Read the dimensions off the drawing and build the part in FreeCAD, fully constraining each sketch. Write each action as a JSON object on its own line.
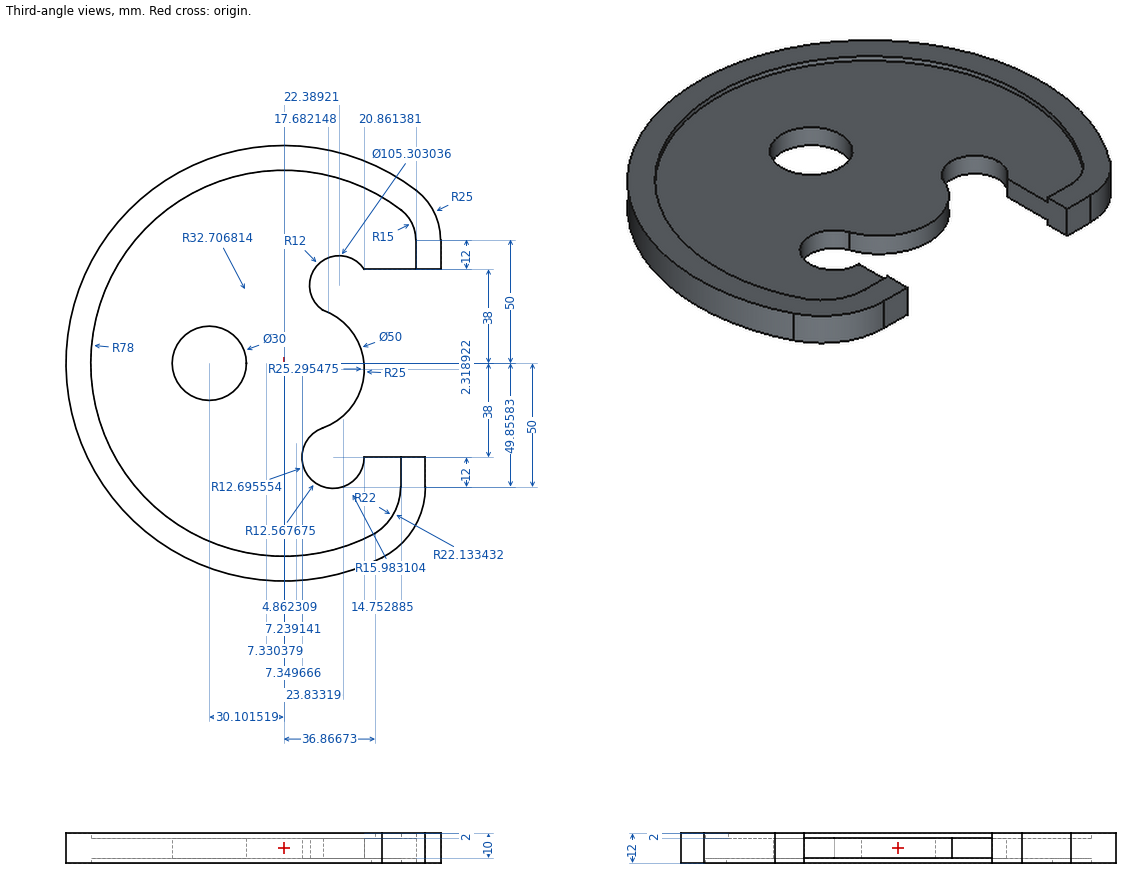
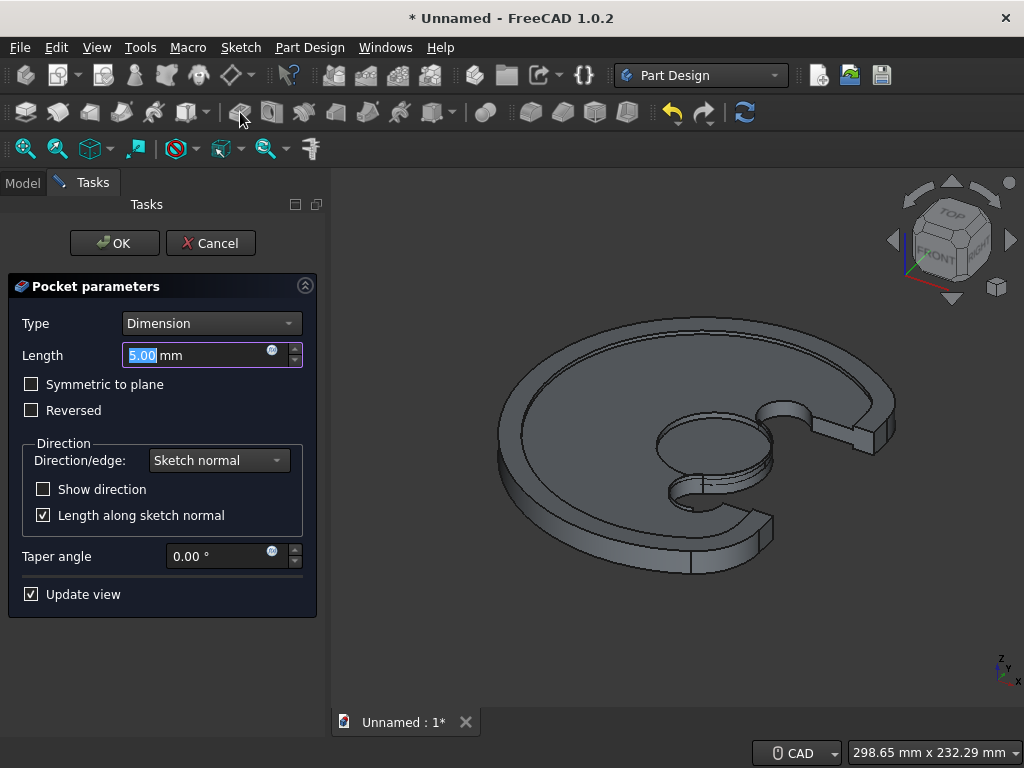
{"action": "type", "text": "2"}
{"action": "key", "text": "Tab"}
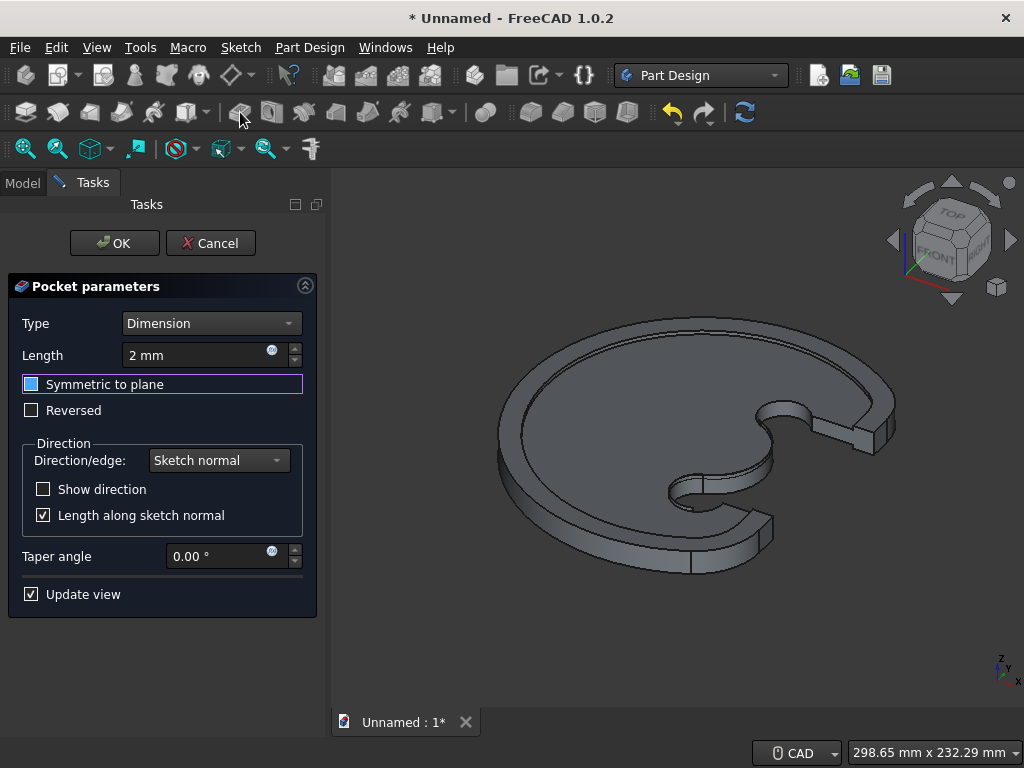
{"action": "left_click", "coordinate": [115, 243]}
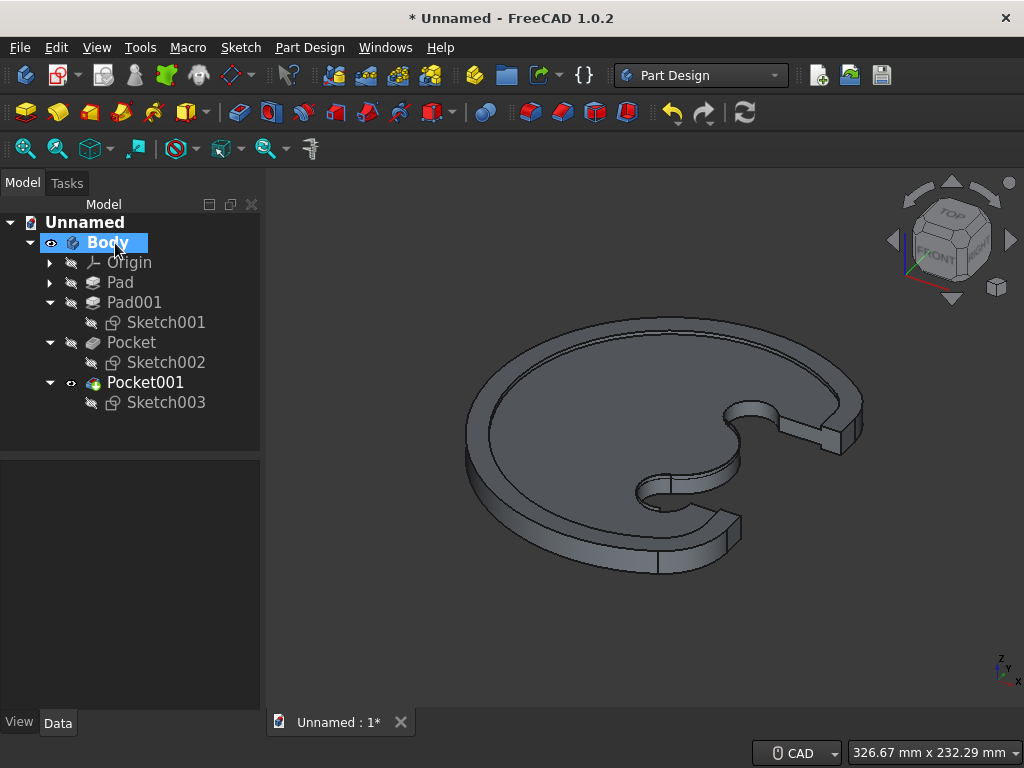
{"action": "left_click", "coordinate": [607, 416]}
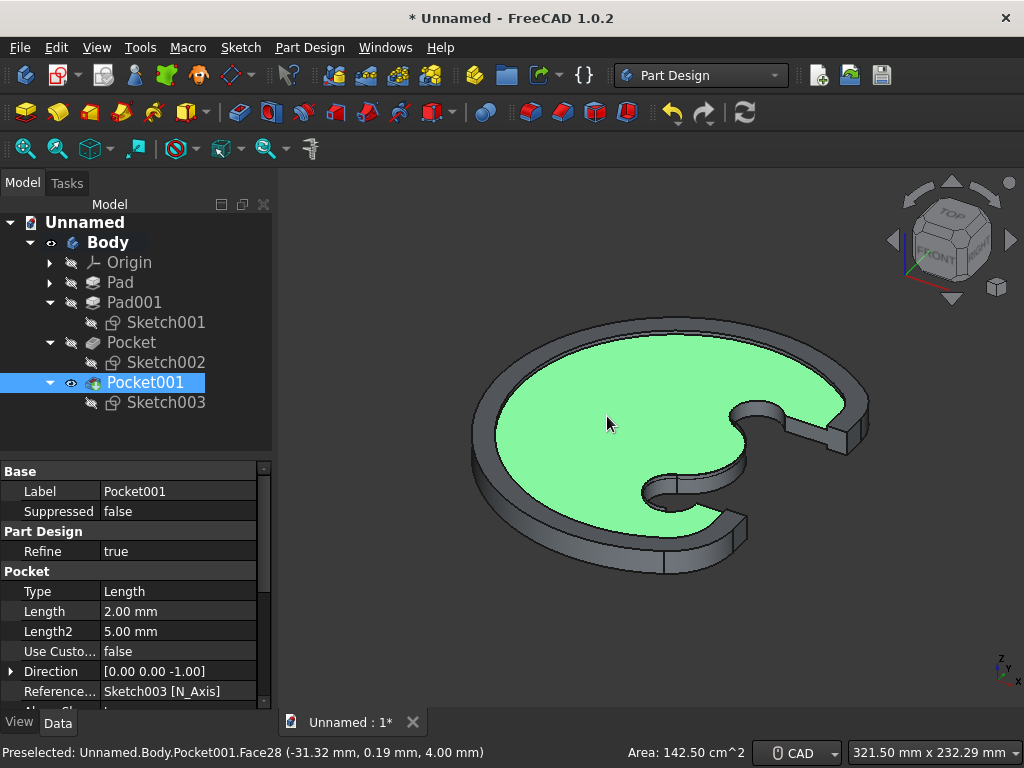
{"action": "left_click", "coordinate": [58, 76]}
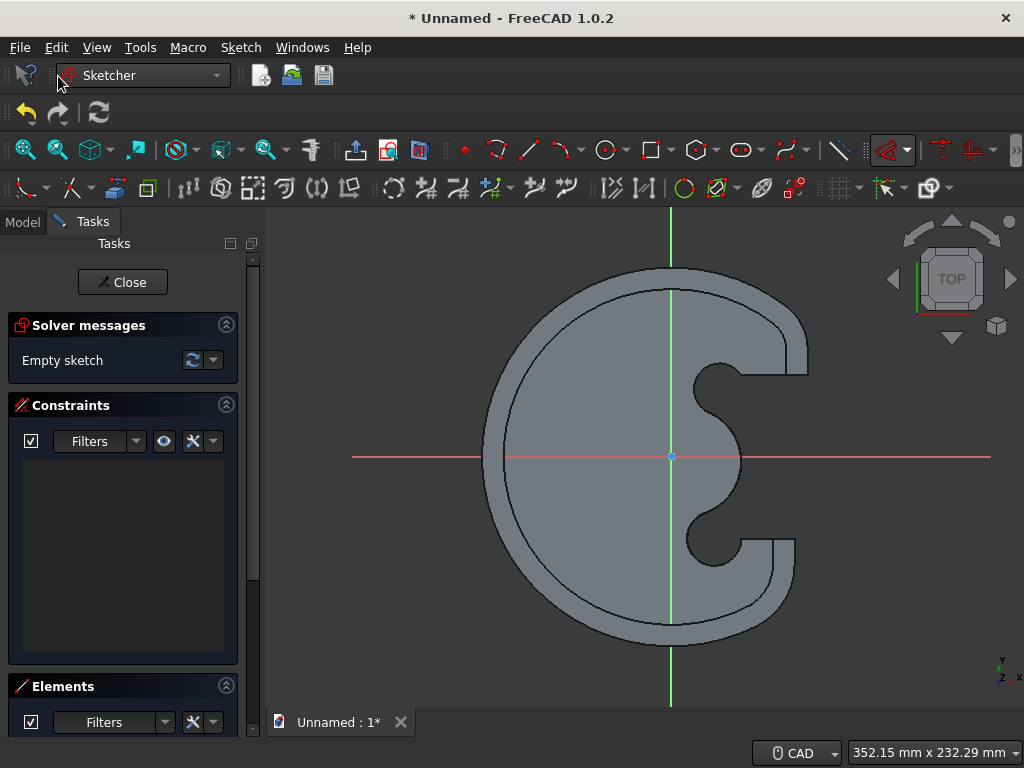
{"action": "scroll", "coordinate": [816, 512], "scroll_direction": "up", "scroll_amount": 3}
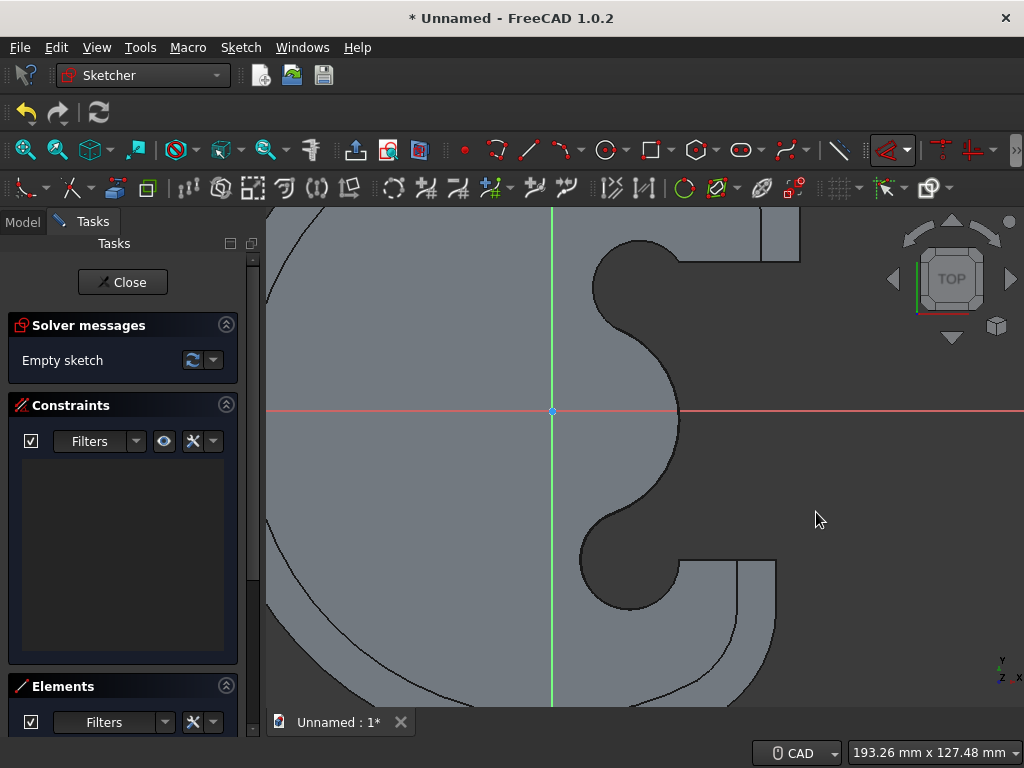
{"action": "key", "text": "g 3 a"}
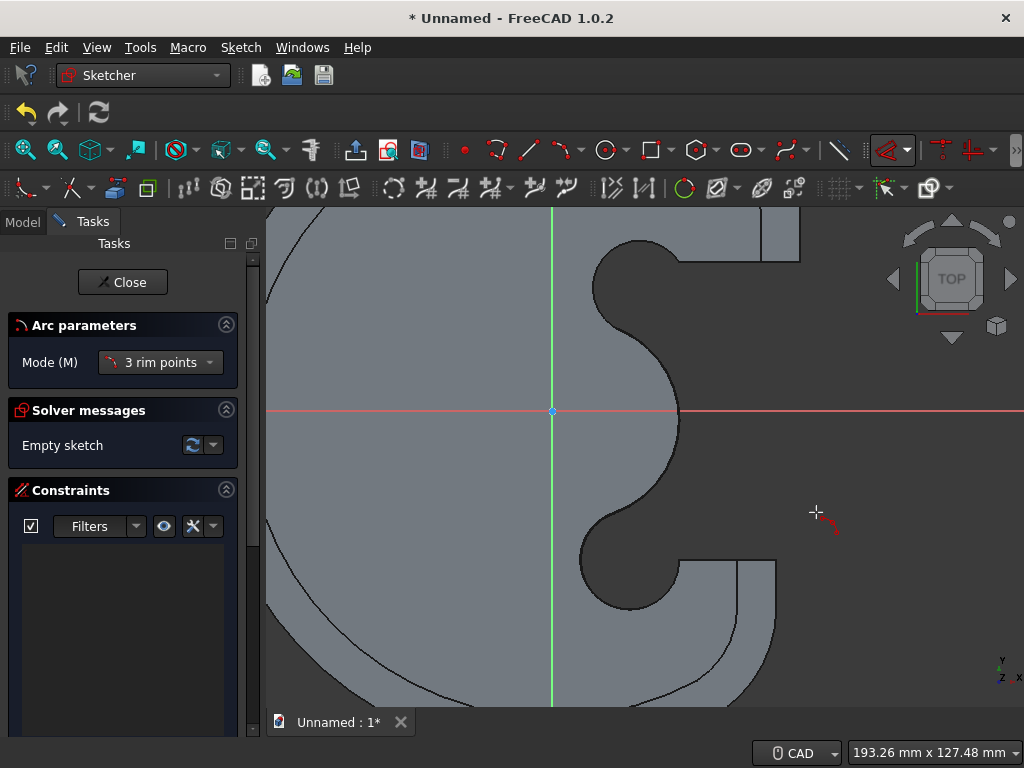
{"action": "left_click", "coordinate": [646, 499]}
{"action": "left_click", "coordinate": [571, 538]}
{"action": "left_click", "coordinate": [492, 298]}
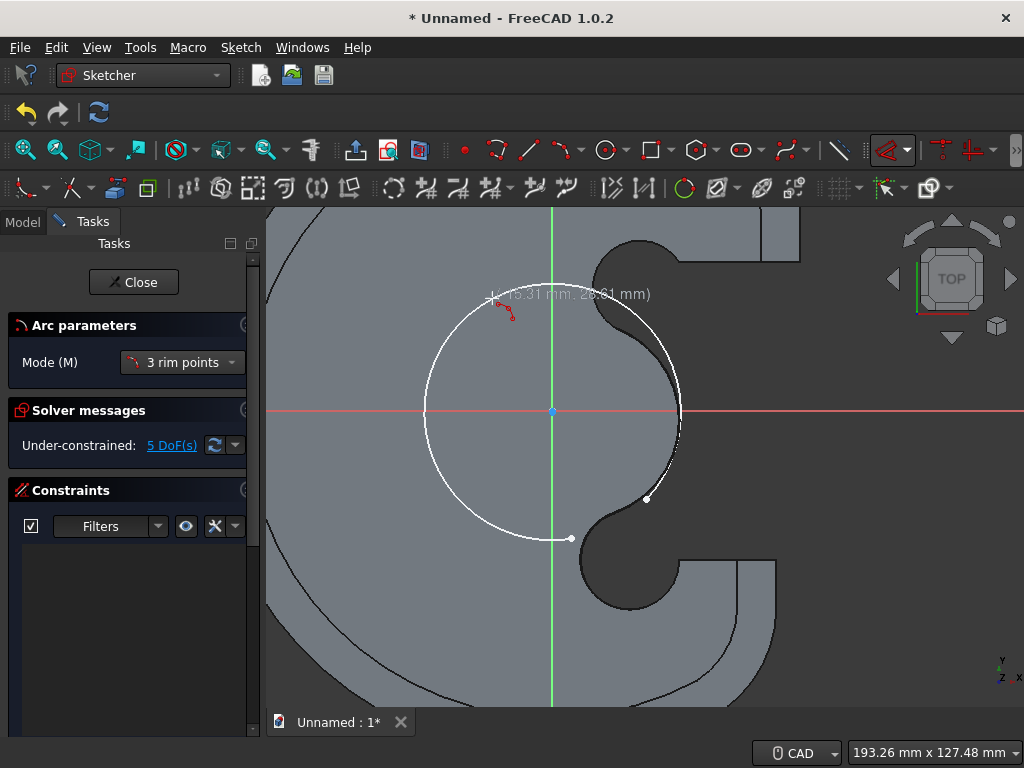
{"action": "left_click", "coordinate": [571, 539]}
{"action": "left_click", "coordinate": [646, 500]}
{"action": "left_click", "coordinate": [659, 615]}
{"action": "key", "text": "Escape"}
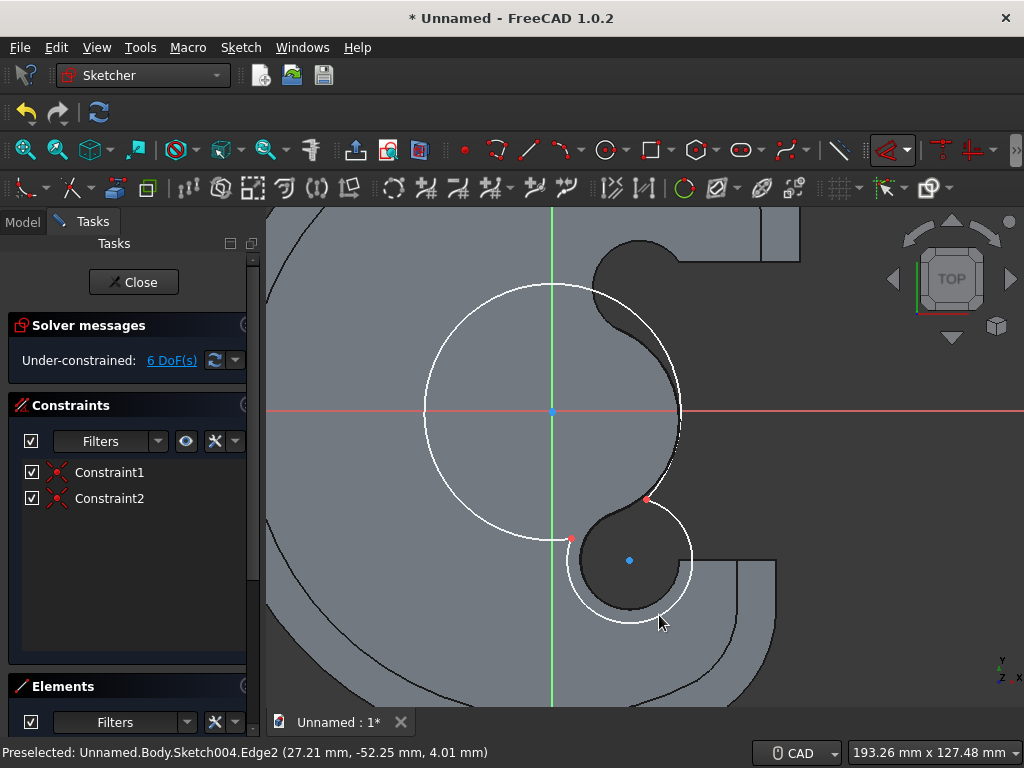
{"action": "left_click_drag", "start_coordinate": [542, 401], "coordinate": [563, 422]}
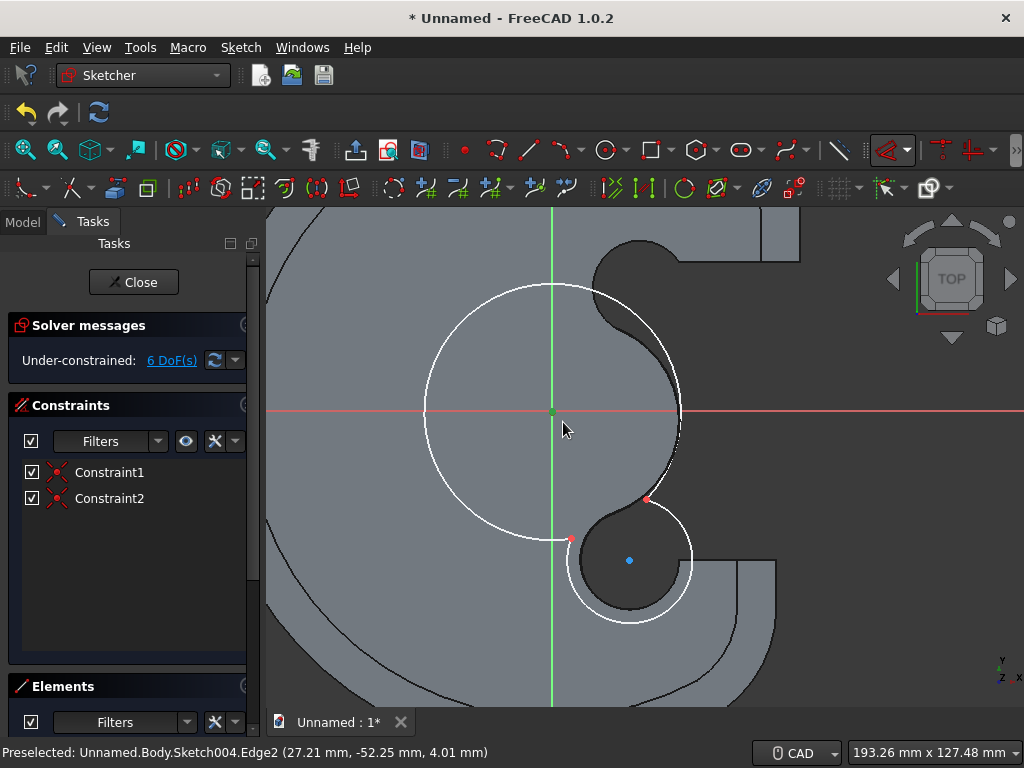
{"action": "left_click", "coordinate": [942, 150]}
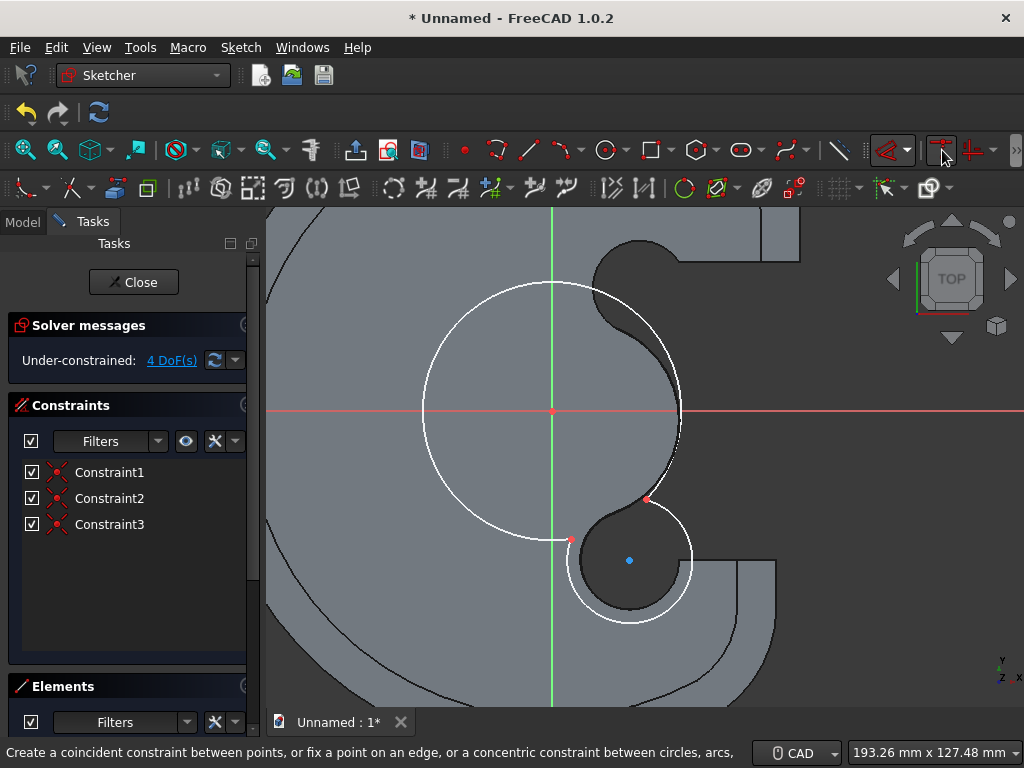
{"action": "left_click", "coordinate": [630, 308]}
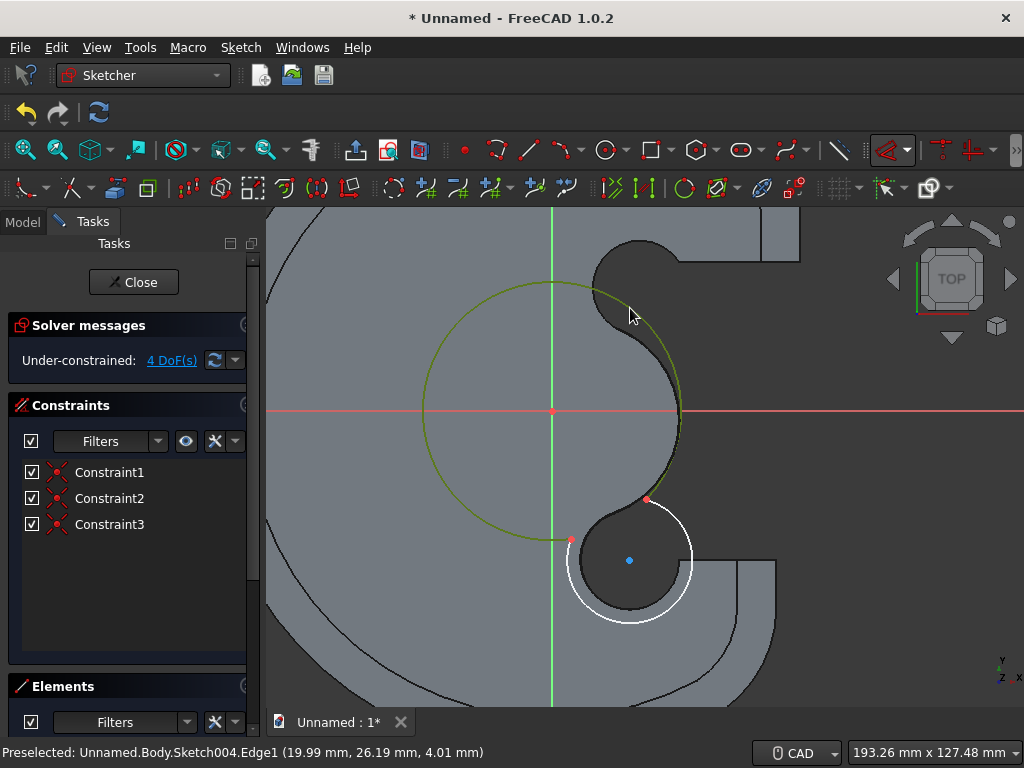
{"action": "key", "text": "k r"}